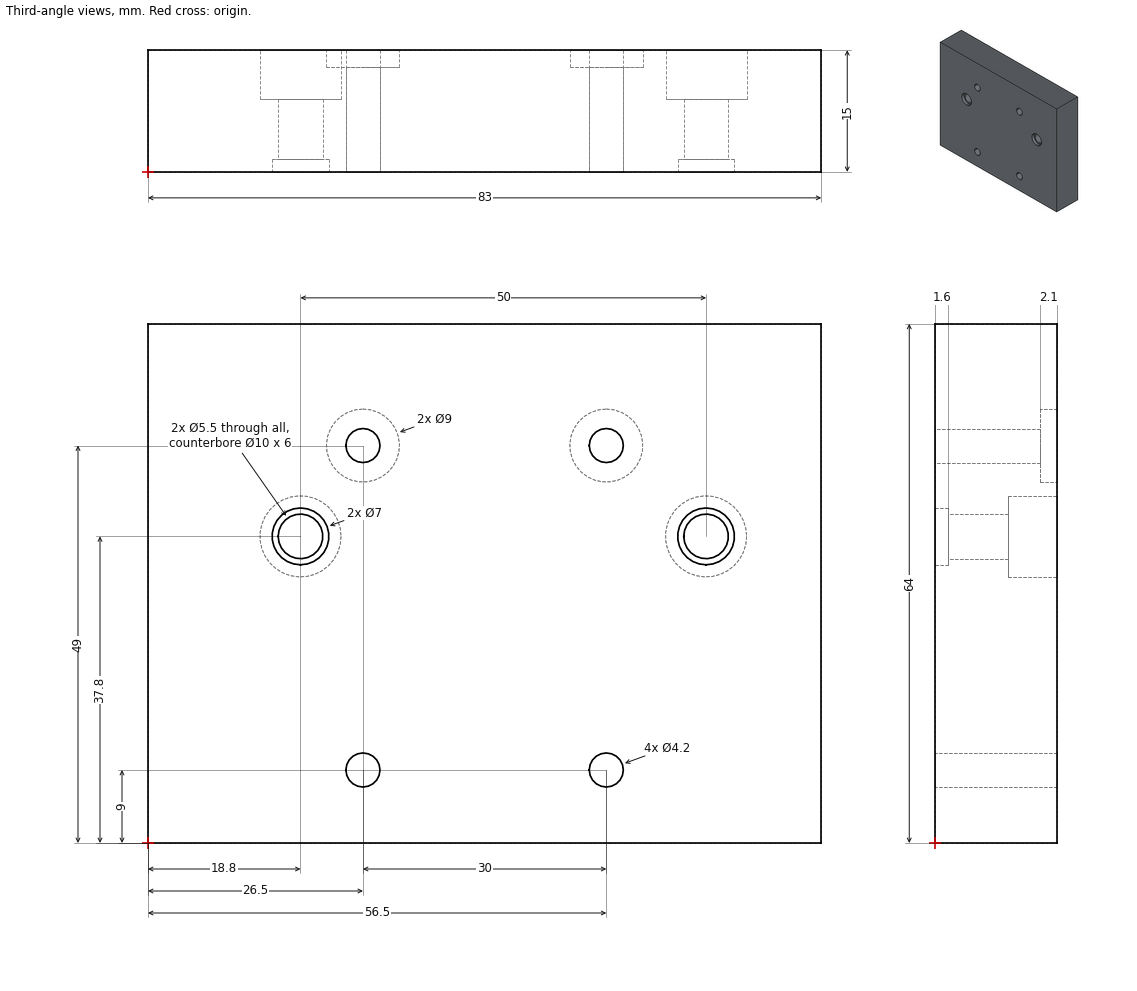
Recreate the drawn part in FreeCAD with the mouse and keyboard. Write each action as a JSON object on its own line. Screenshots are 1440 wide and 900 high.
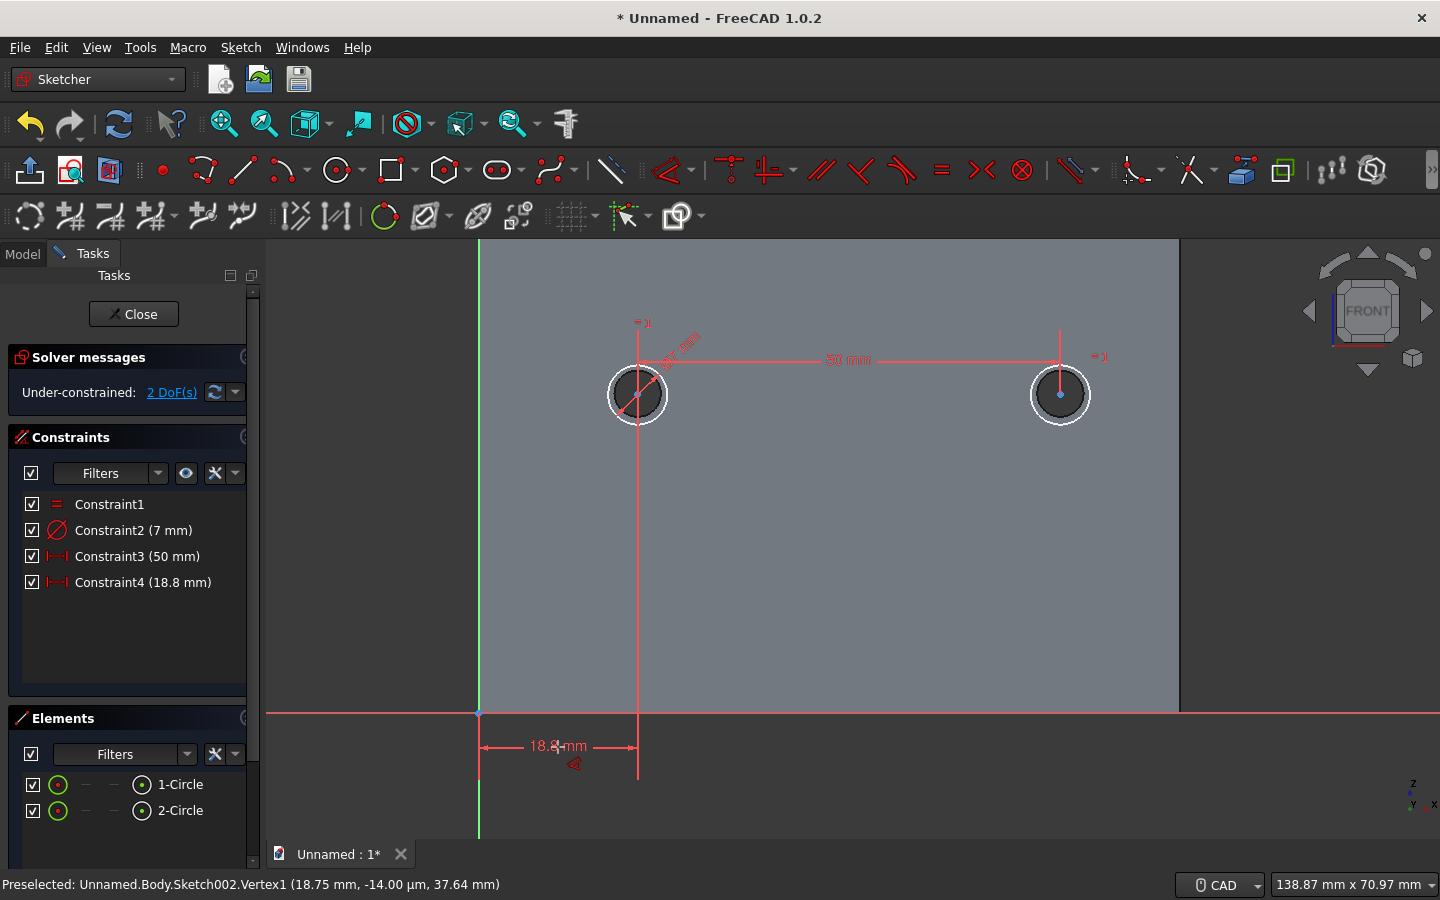
{"action": "left_click", "coordinate": [638, 395]}
{"action": "left_click", "coordinate": [445, 554]}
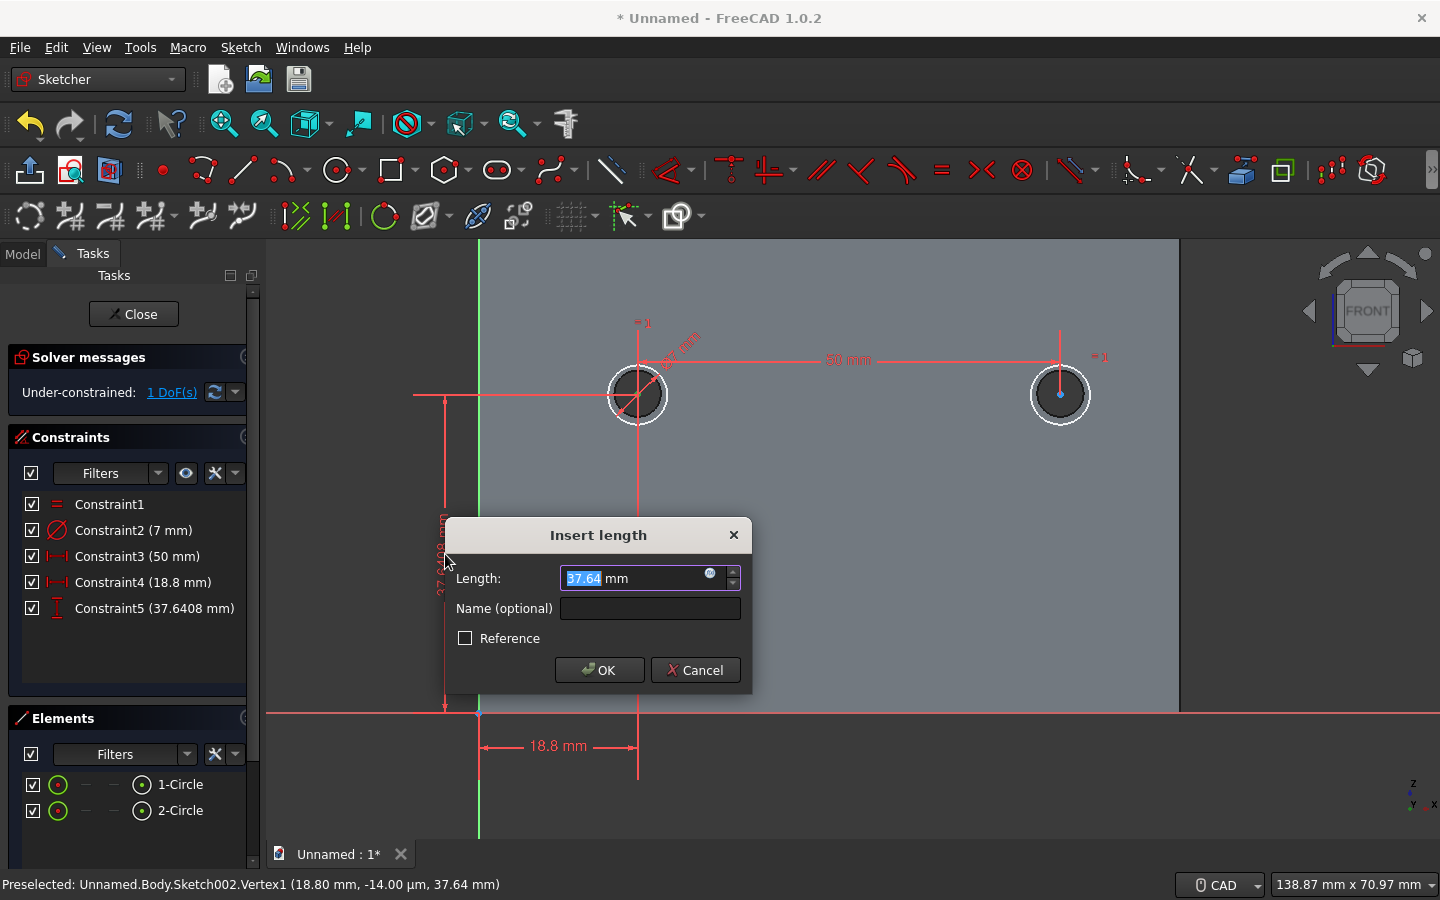
{"action": "type", "text": "37.8"}
{"action": "key", "text": "Return"}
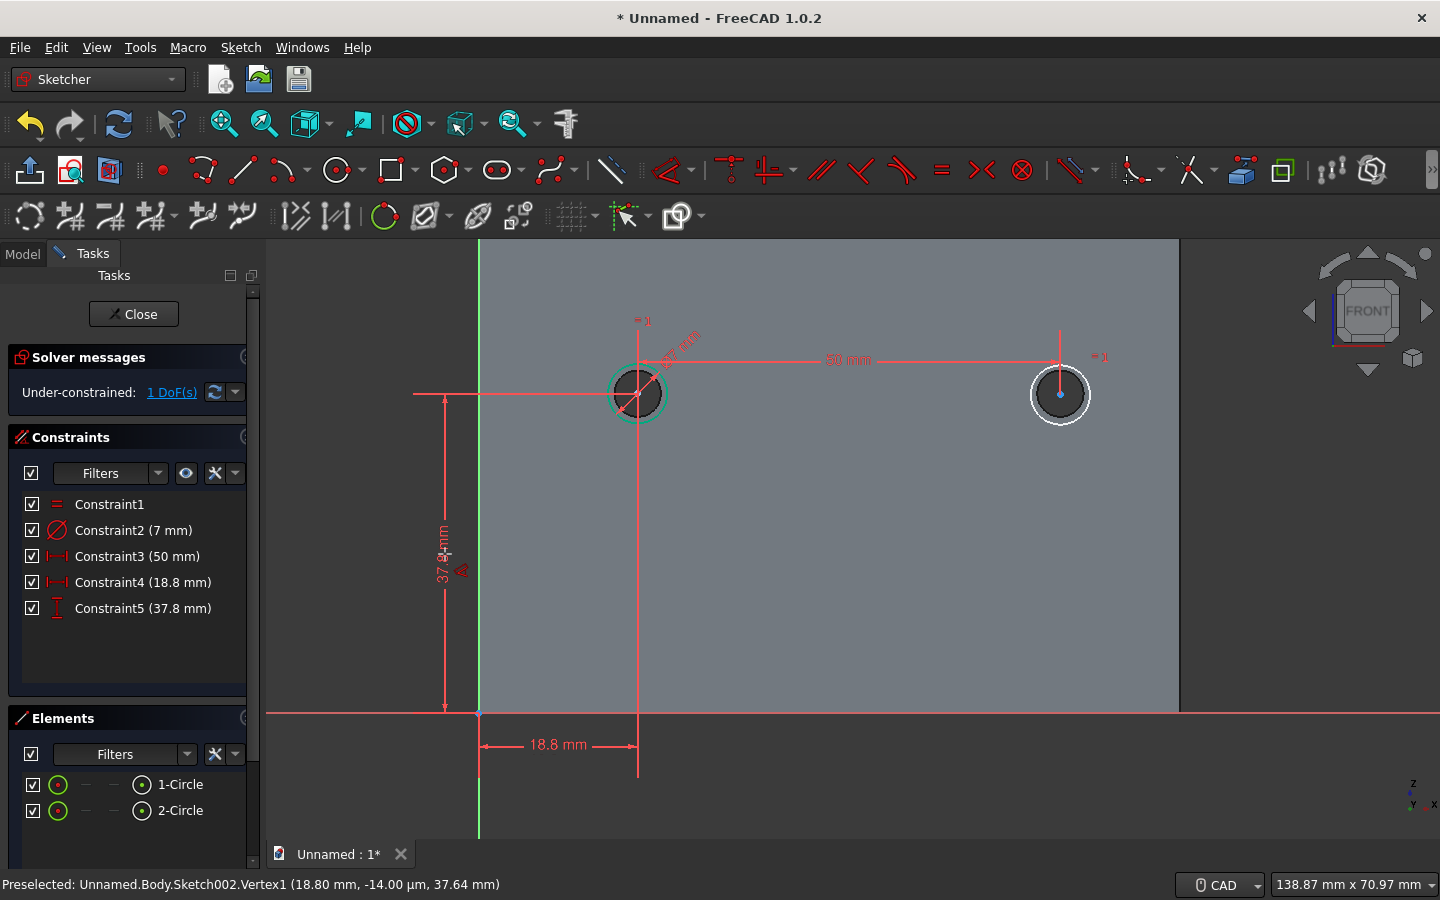
{"action": "left_click", "coordinate": [1060, 395]}
{"action": "left_click", "coordinate": [445, 481]}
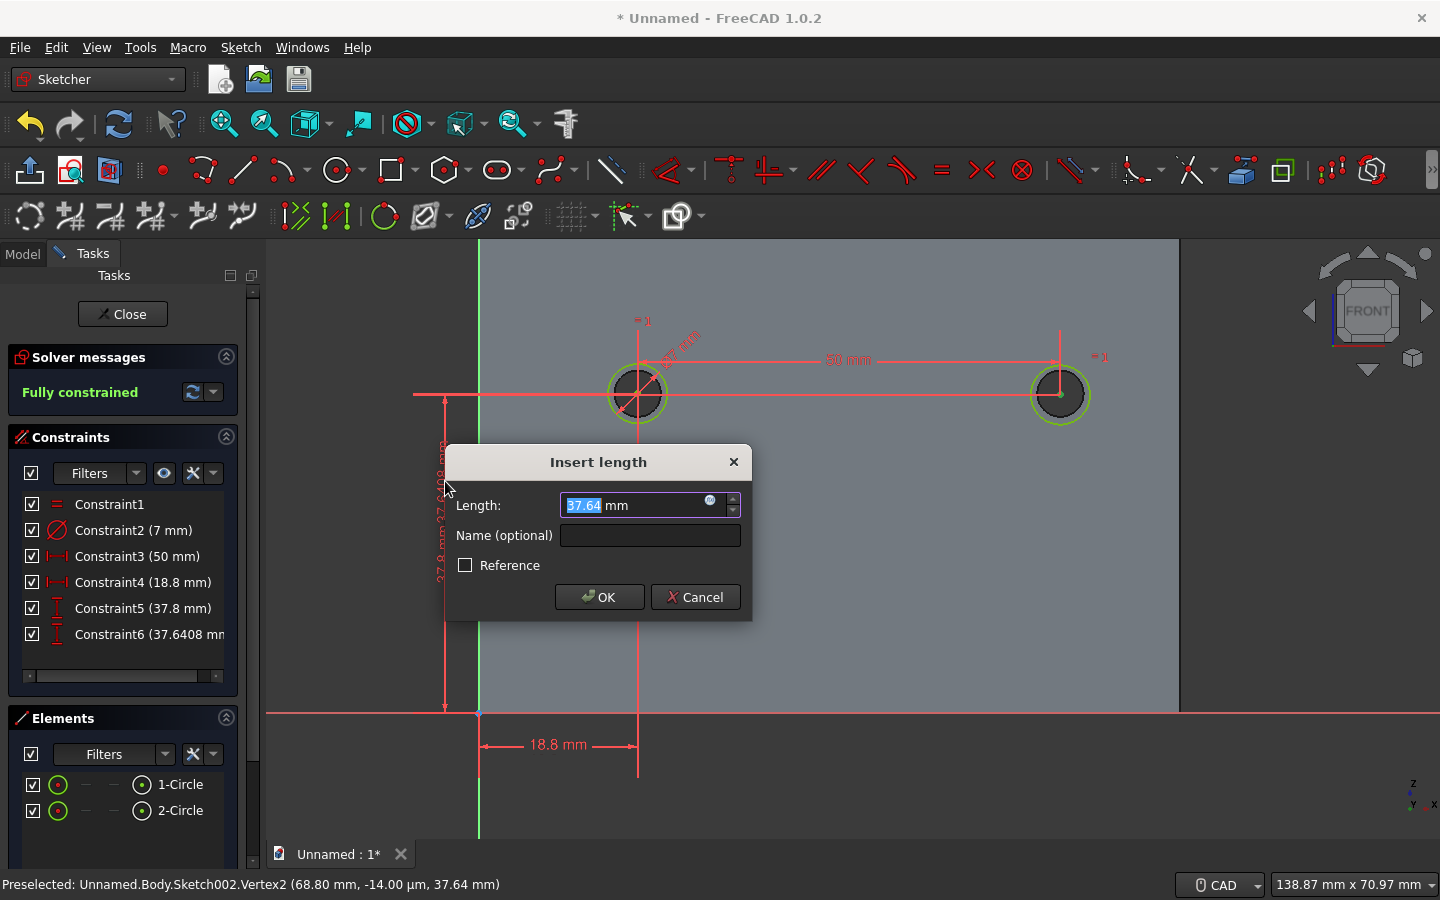
{"action": "type", "text": "37.8"}
{"action": "key", "text": "Return"}
{"action": "key", "text": "Escape"}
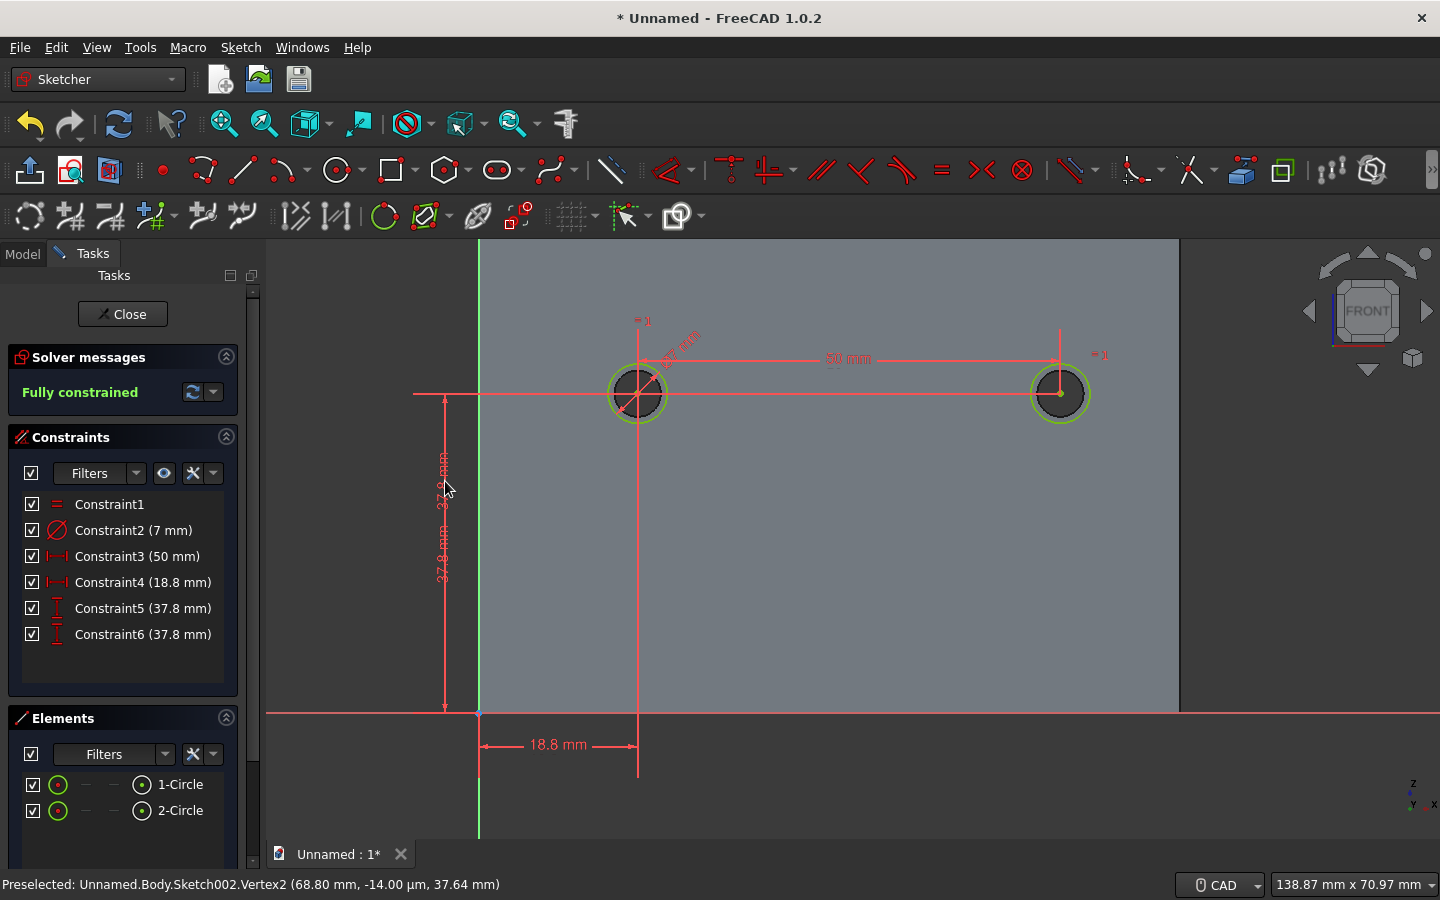
{"action": "left_click", "coordinate": [123, 314]}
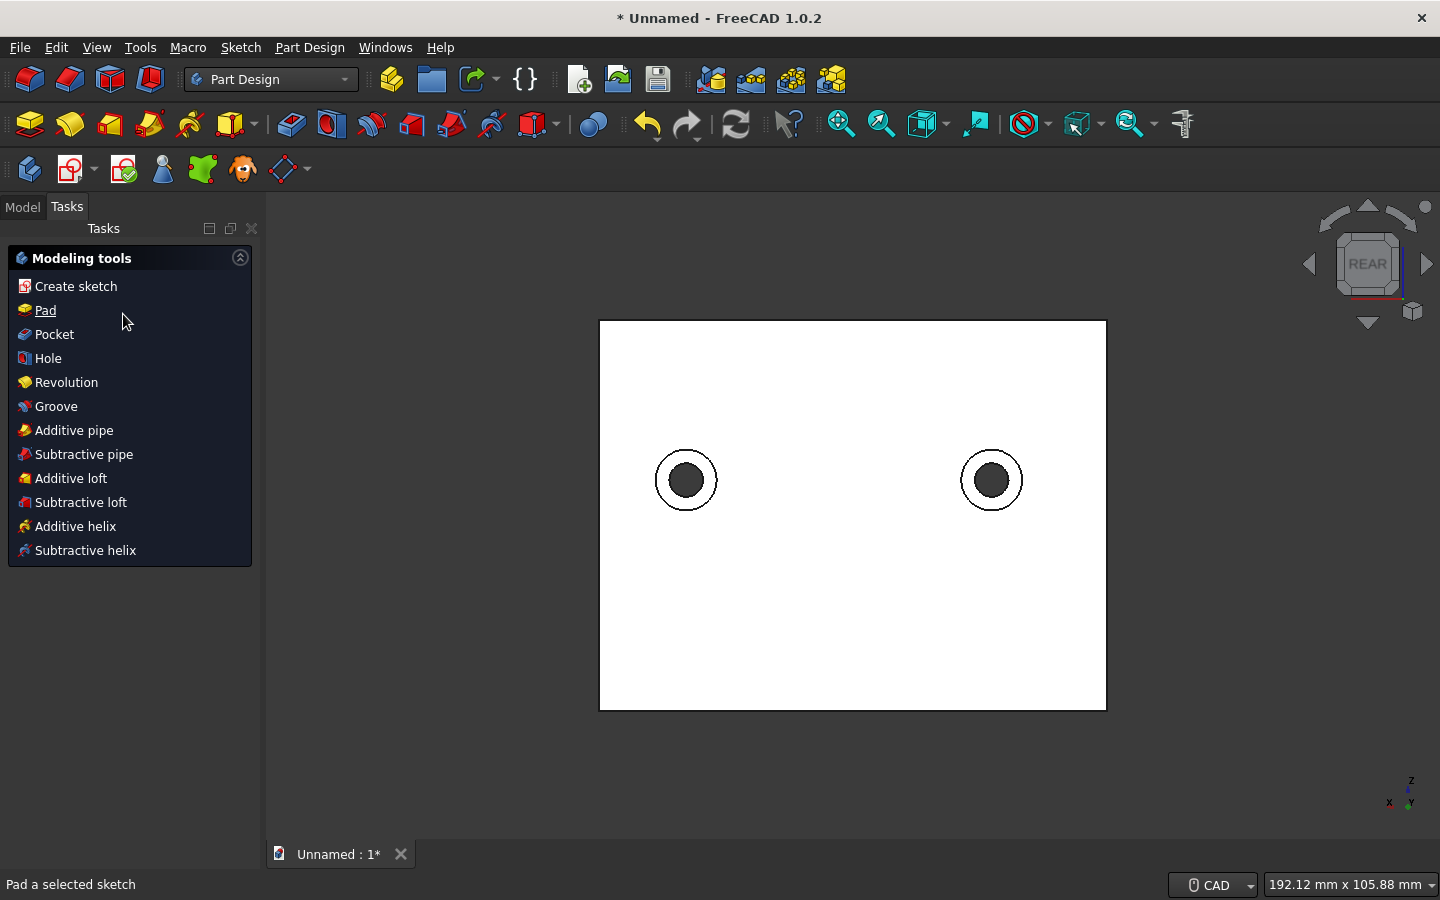
{"action": "left_click", "coordinate": [292, 124]}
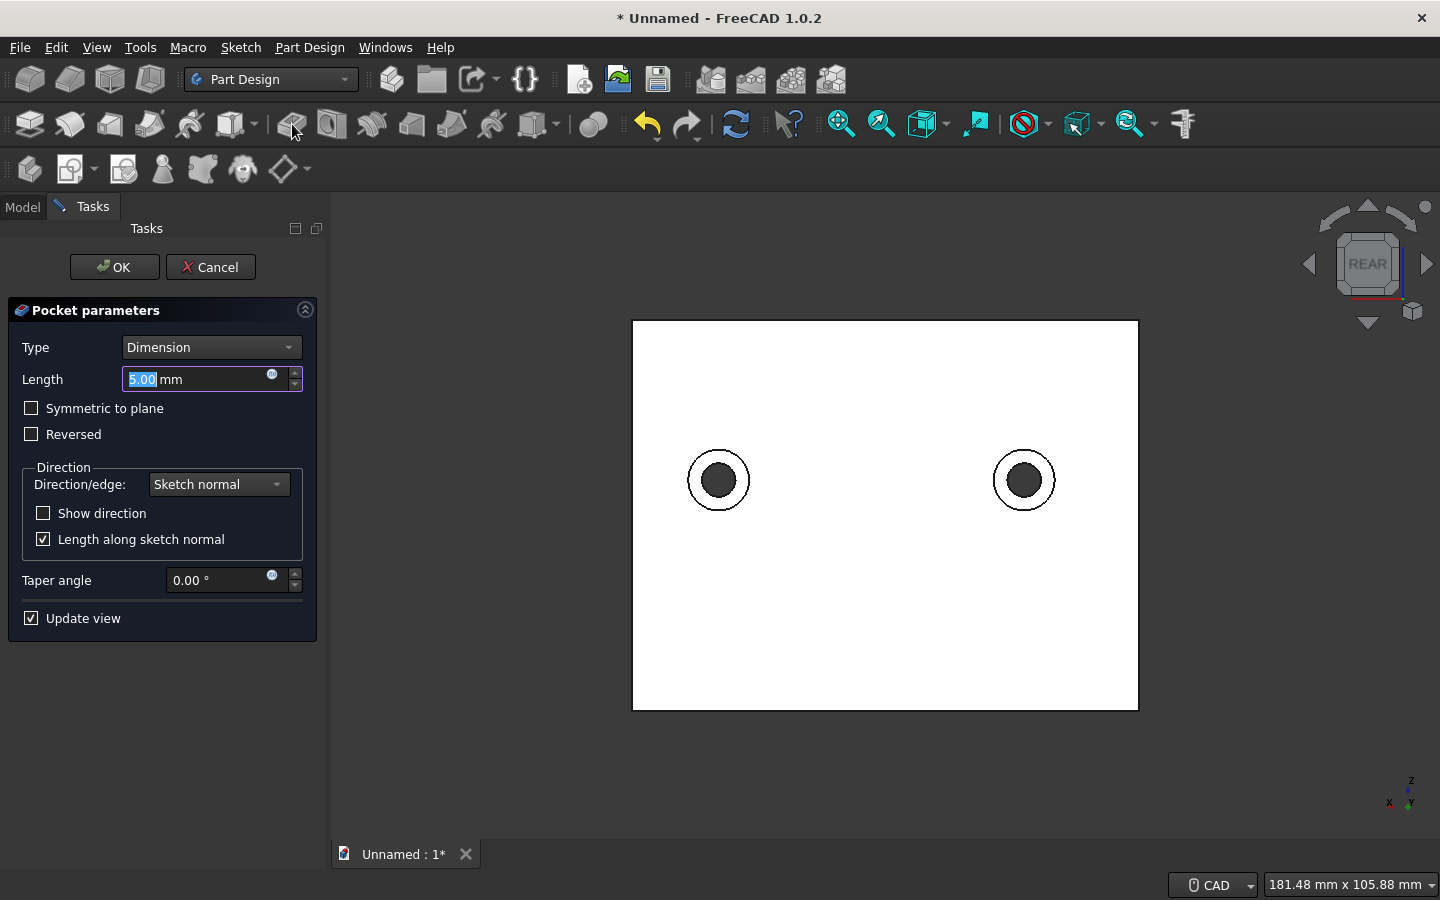
{"action": "type", "text": "1.6"}
{"action": "key", "text": "Tab"}